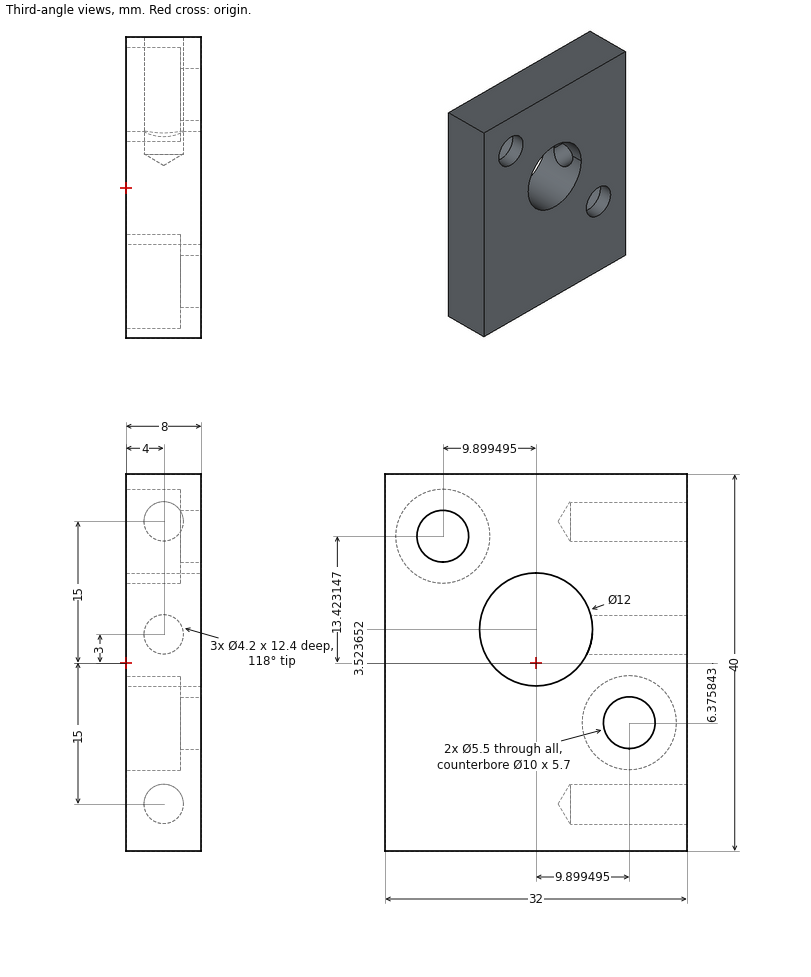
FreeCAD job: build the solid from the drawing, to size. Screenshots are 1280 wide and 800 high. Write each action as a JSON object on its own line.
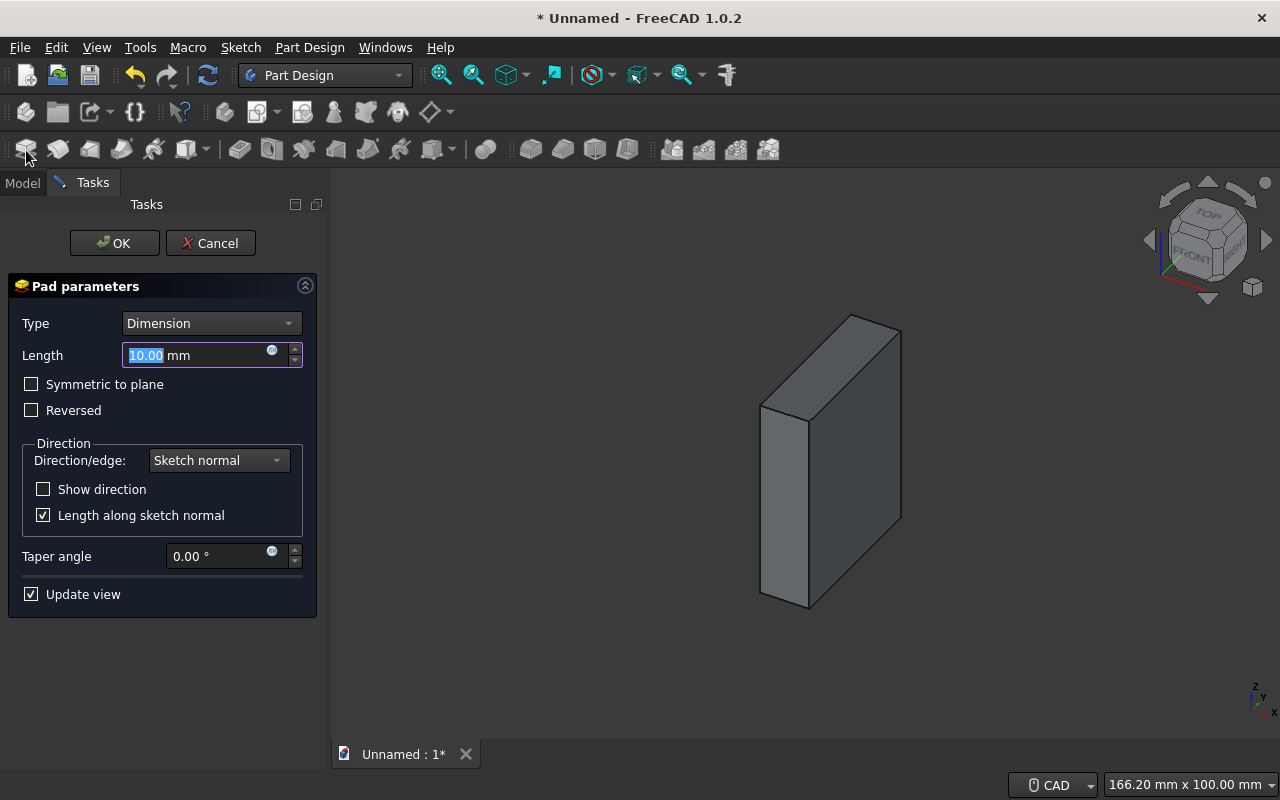
{"action": "type", "text": "8"}
{"action": "key", "text": "Tab"}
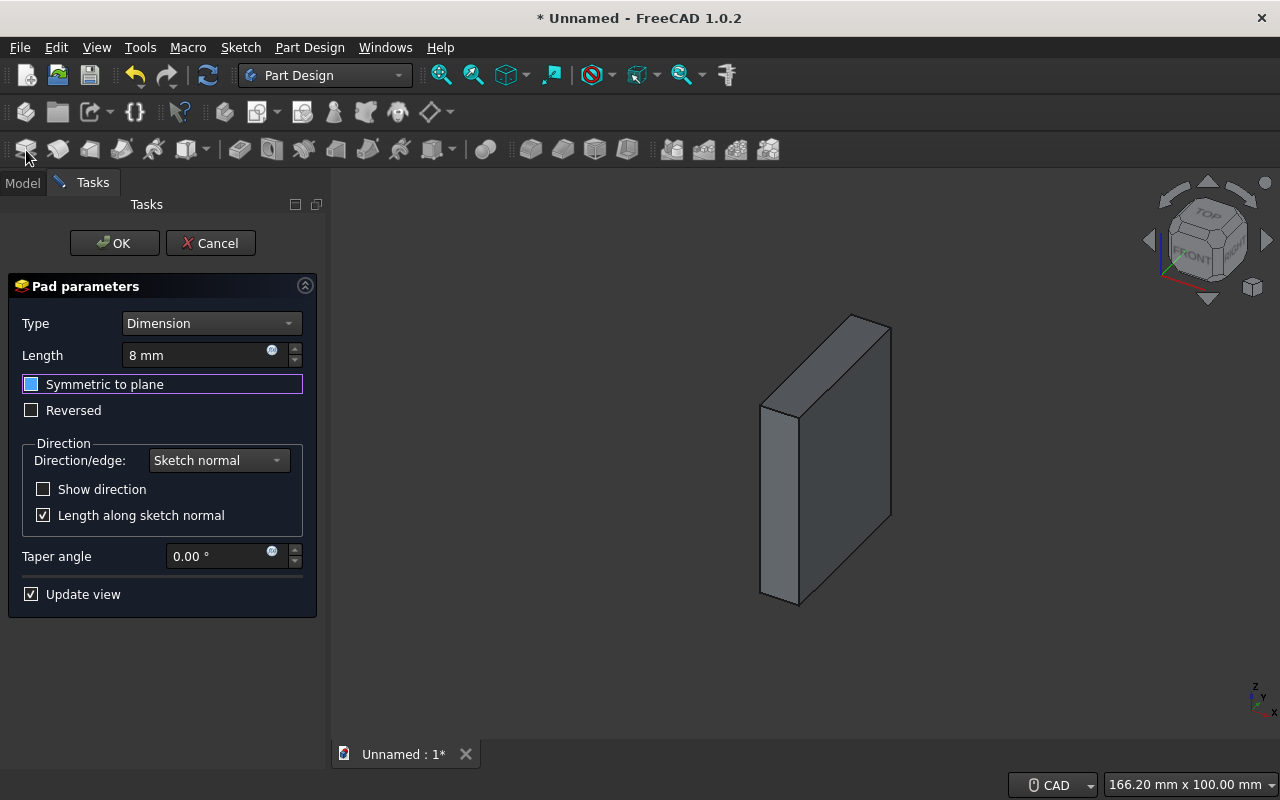
{"action": "left_click", "coordinate": [115, 243]}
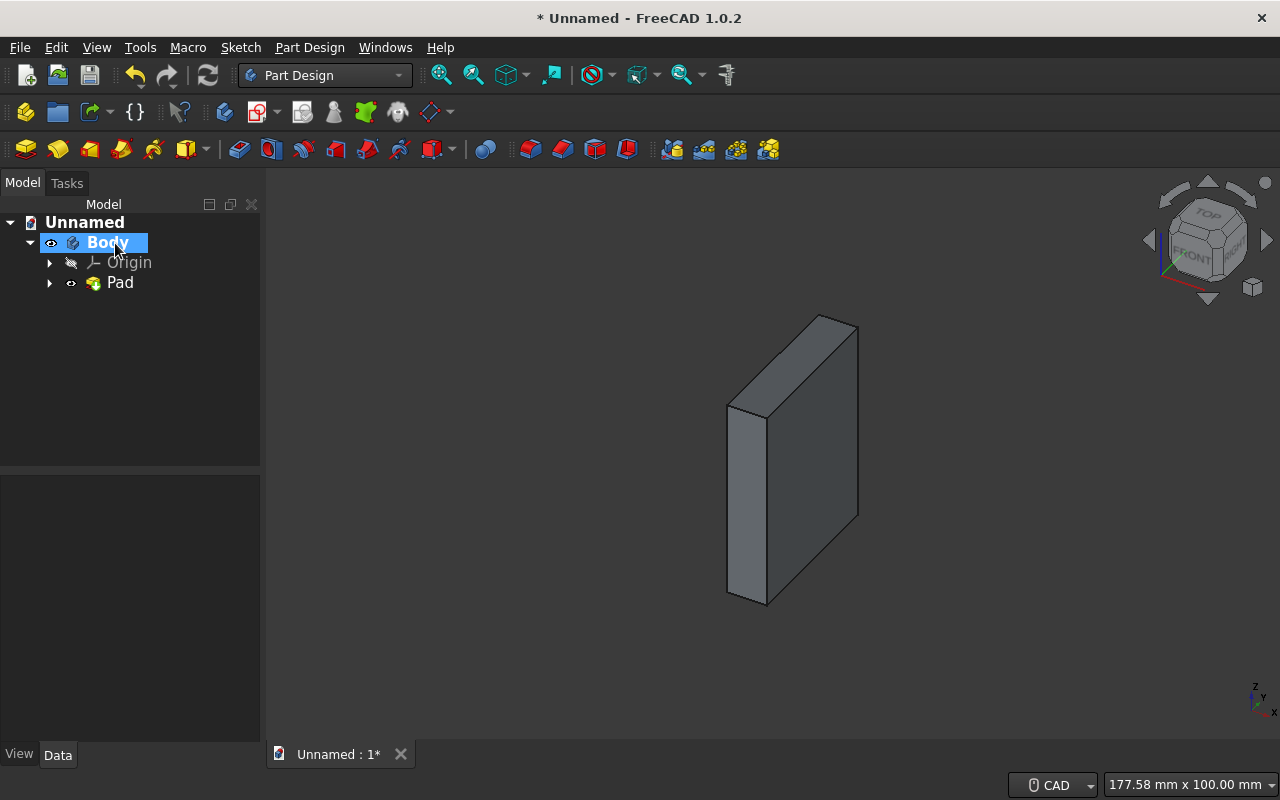
{"action": "left_click", "coordinate": [258, 112]}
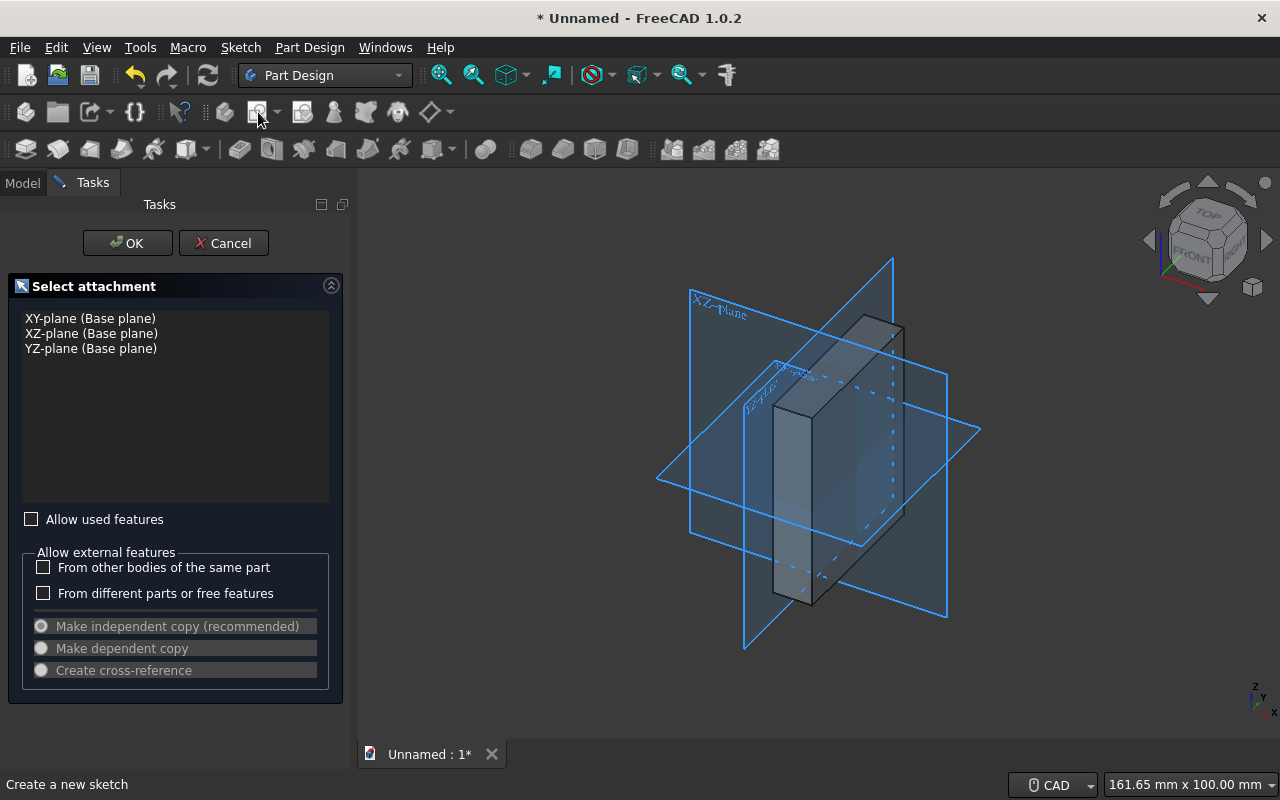
{"action": "left_click", "coordinate": [82, 348]}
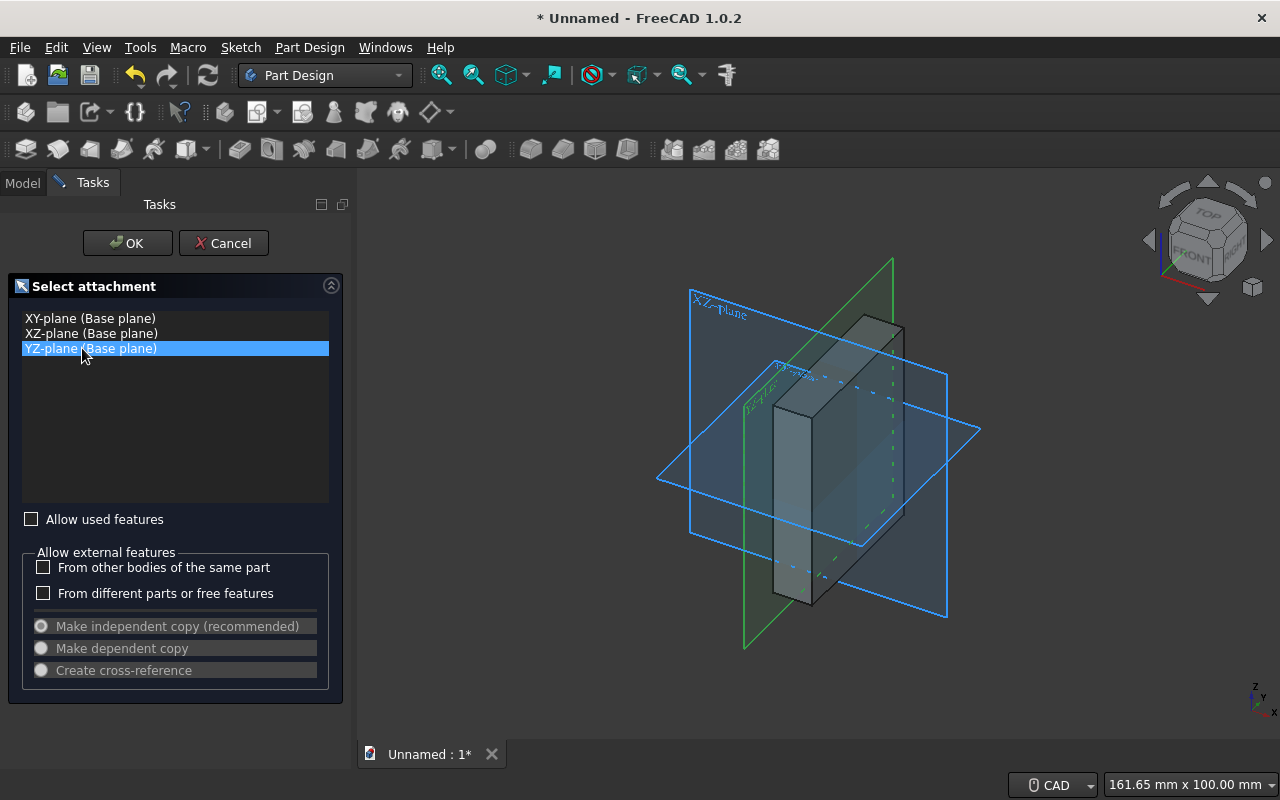
{"action": "left_click", "coordinate": [128, 243]}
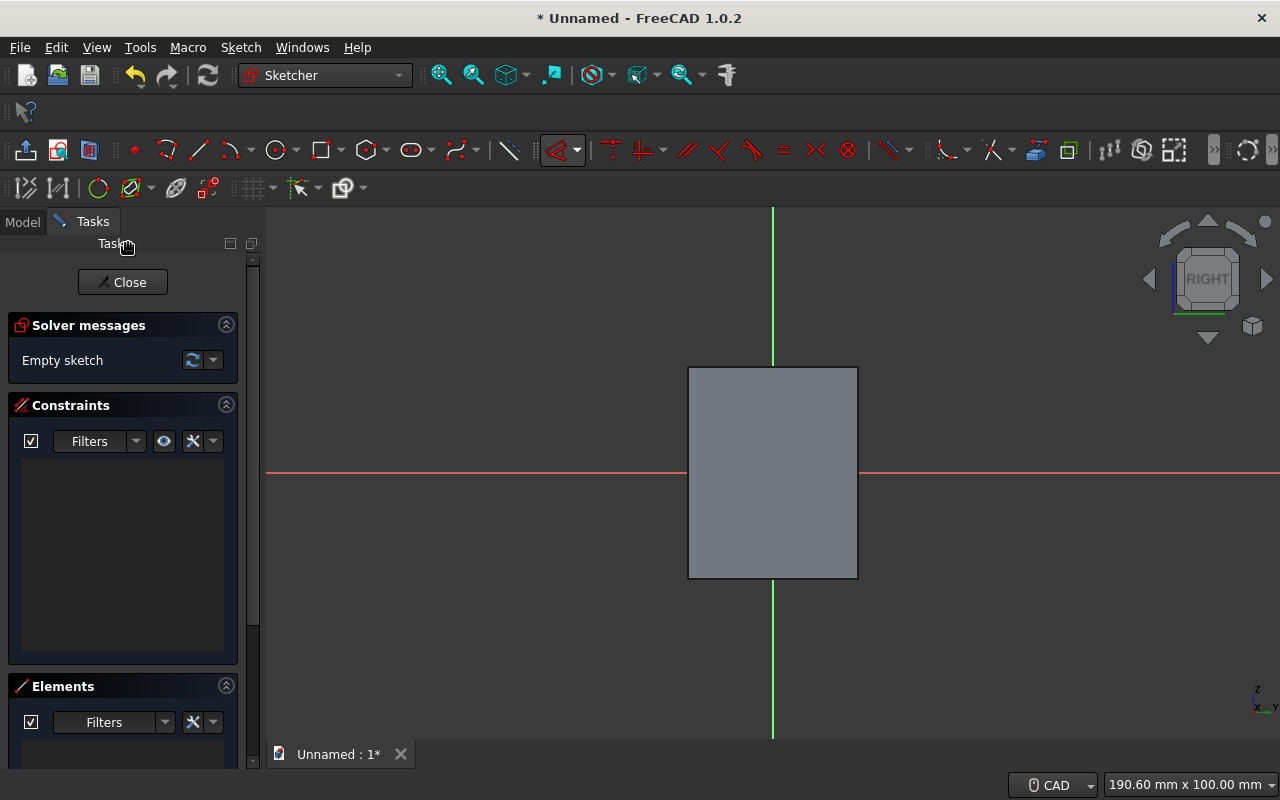
{"action": "key", "text": "q s"}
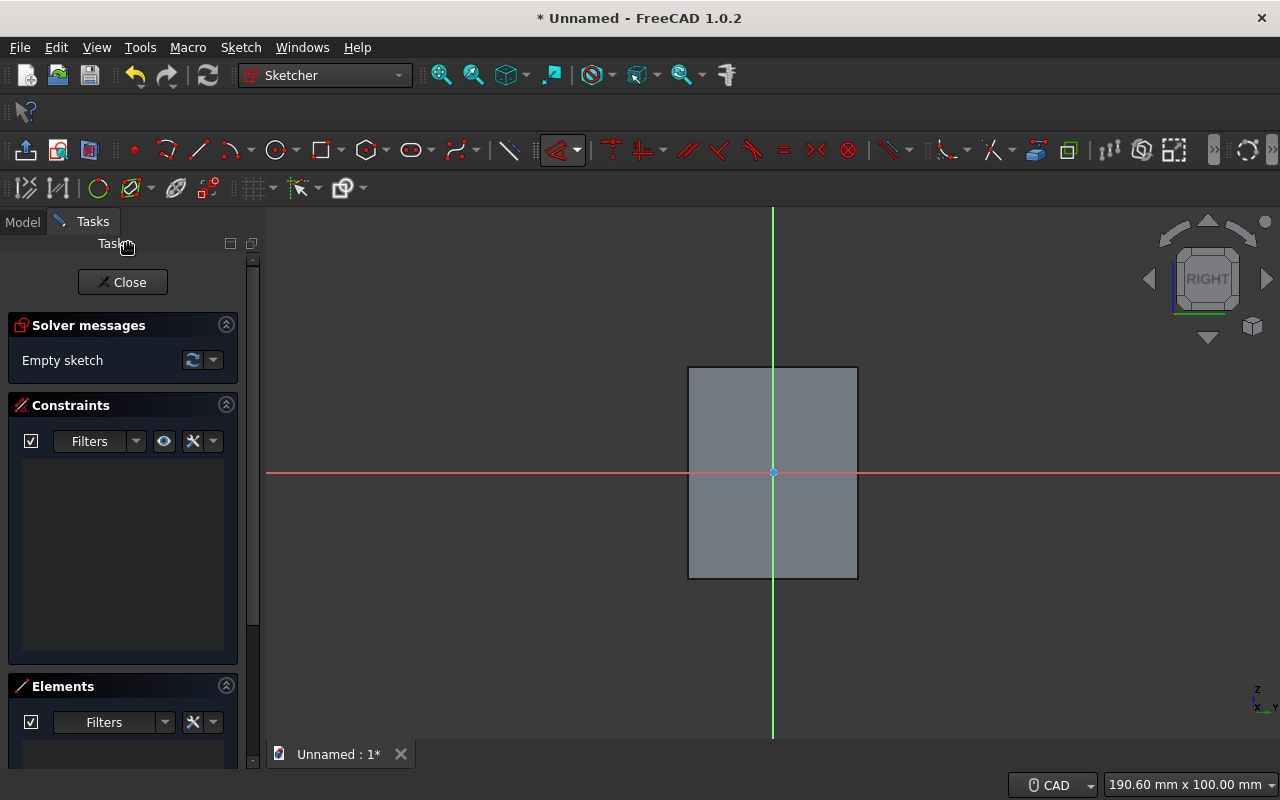
{"action": "scroll", "coordinate": [790, 450], "scroll_direction": "up", "scroll_amount": 8}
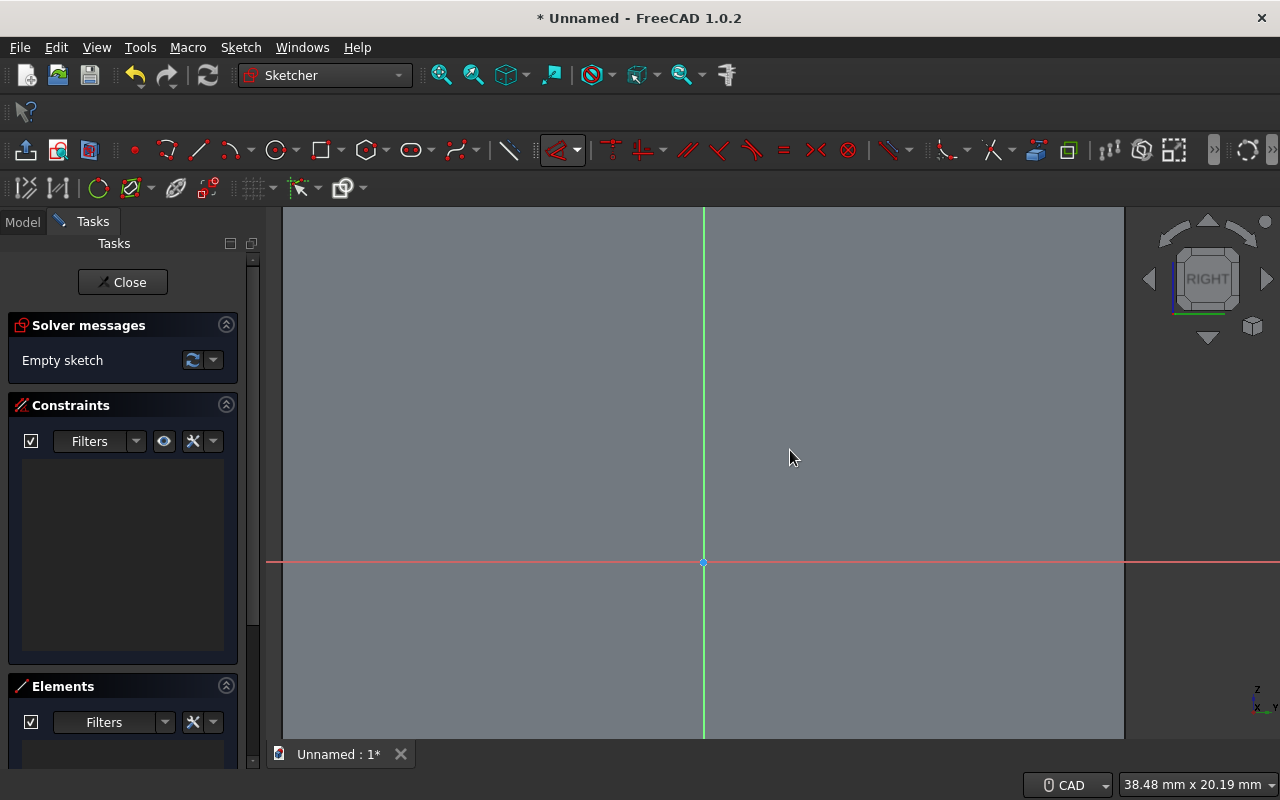
{"action": "key", "text": "g c"}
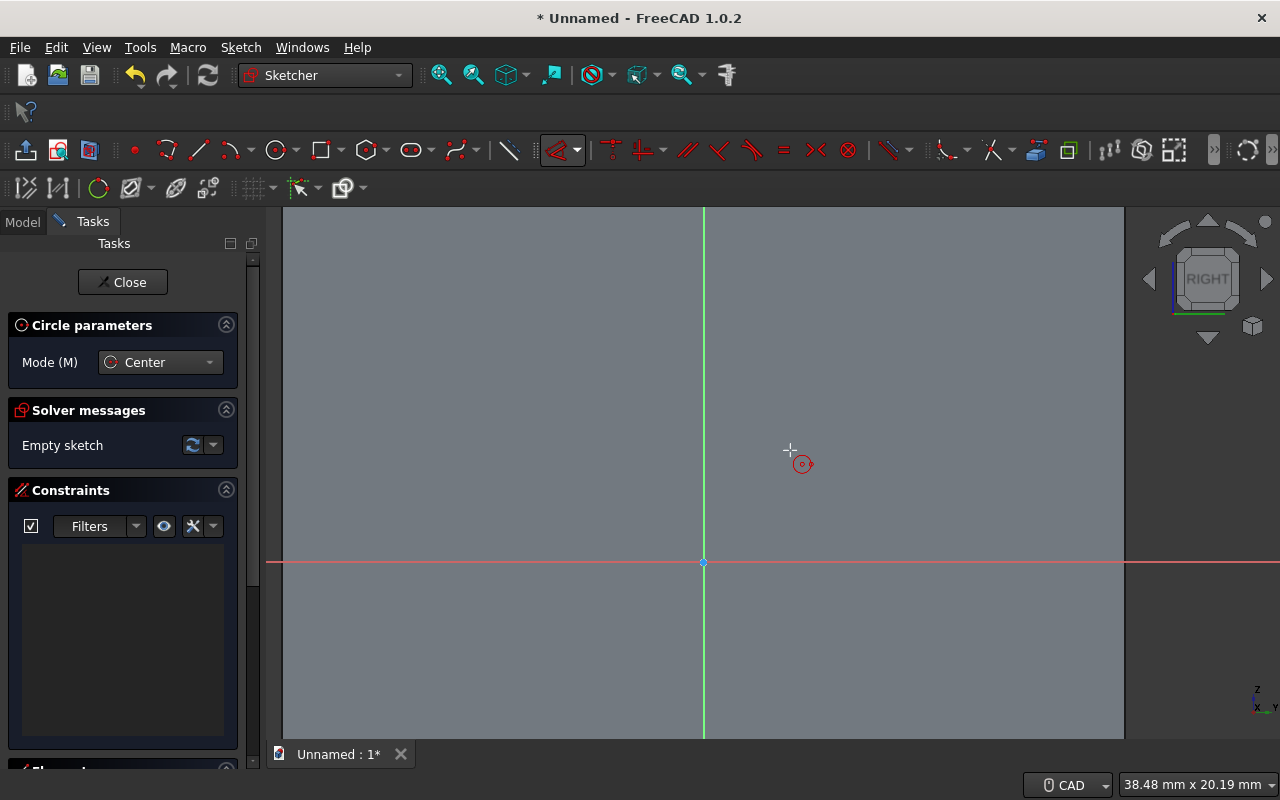
{"action": "left_click", "coordinate": [704, 469]}
{"action": "mouse_move", "coordinate": [816, 357]}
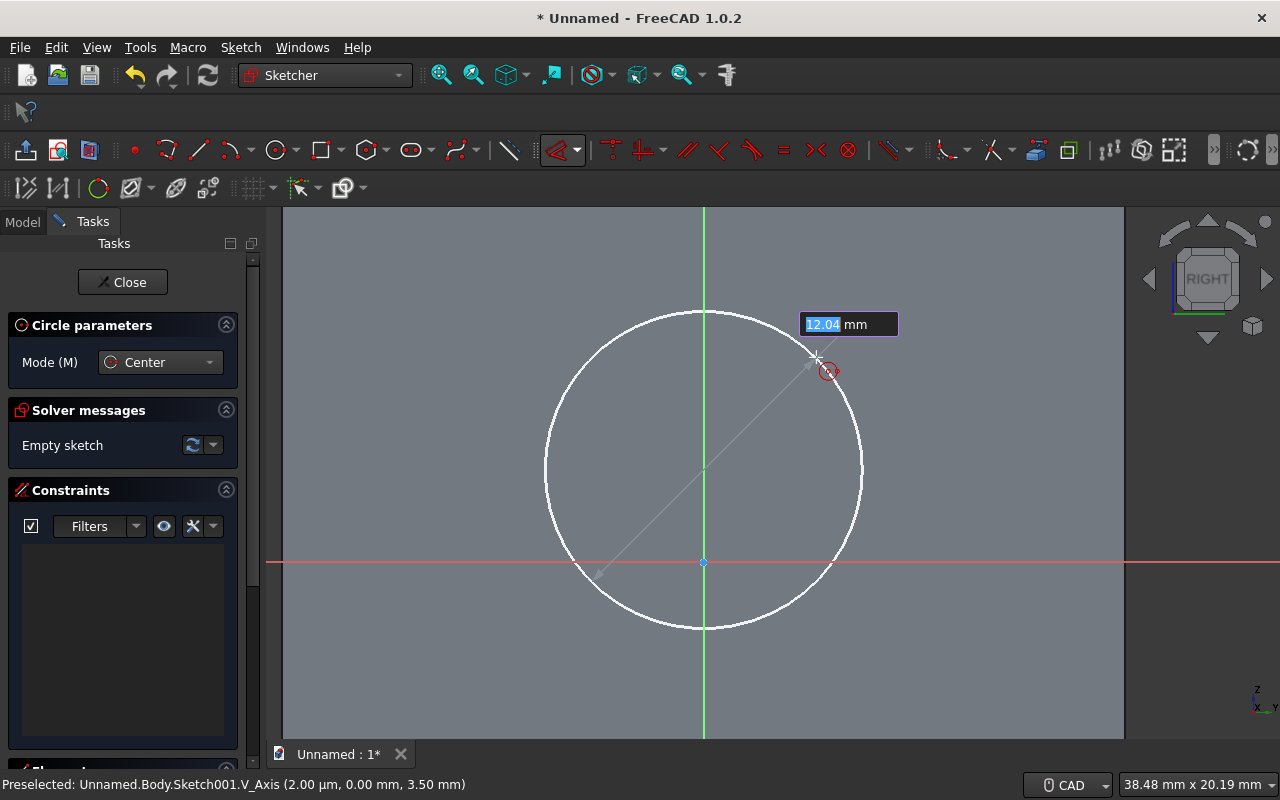
{"action": "type", "text": "12"}
{"action": "key", "text": "Return"}
{"action": "key", "text": "Escape"}